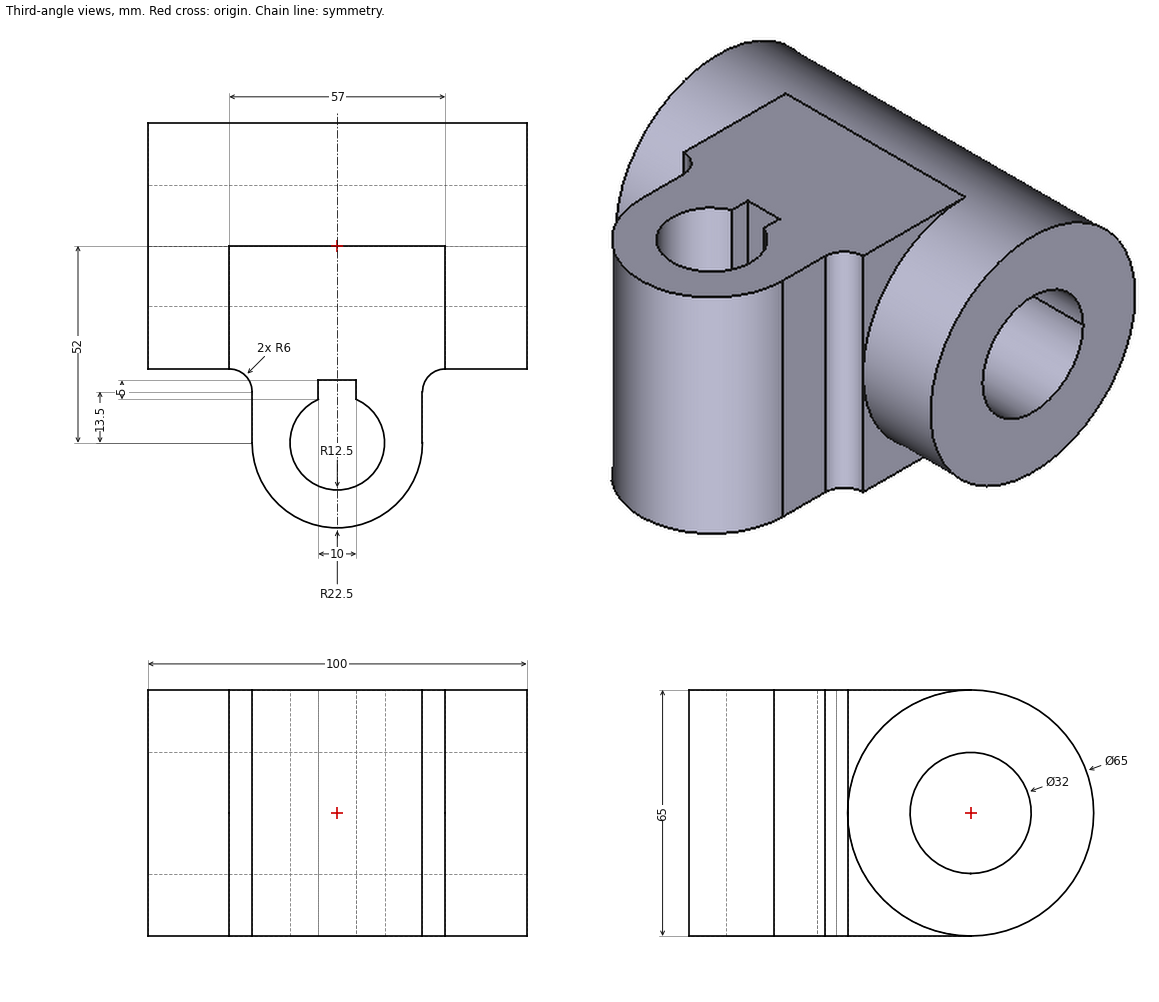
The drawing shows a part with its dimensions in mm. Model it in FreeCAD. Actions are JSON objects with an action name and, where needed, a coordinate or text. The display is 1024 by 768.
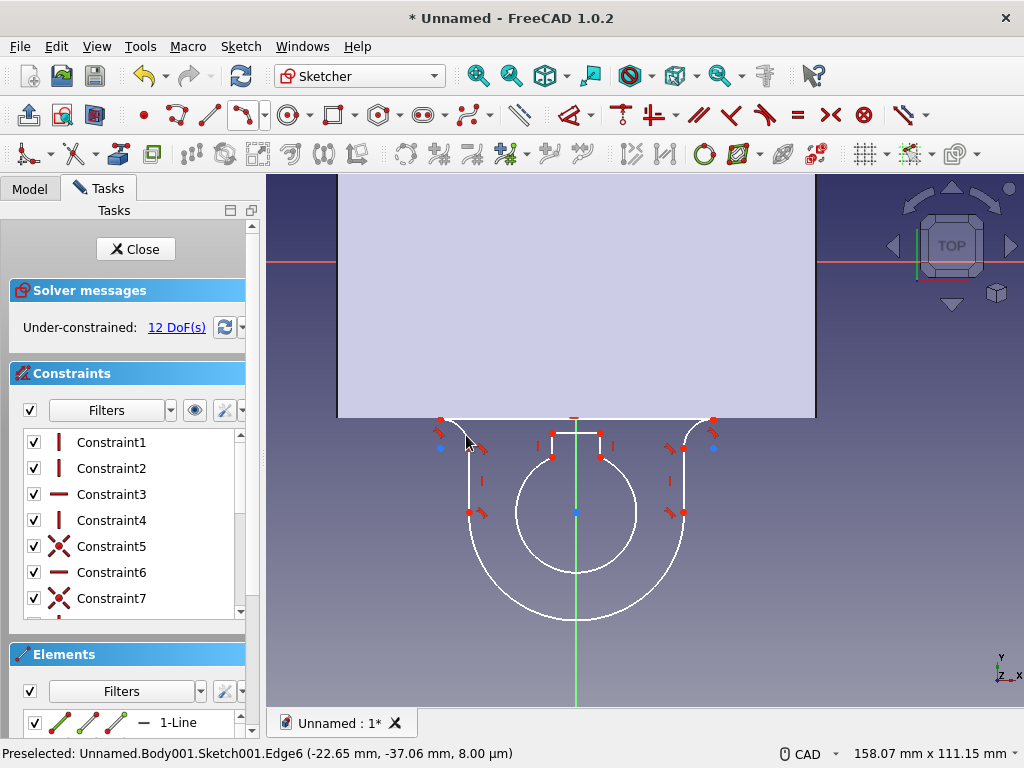
{"action": "left_click", "coordinate": [513, 600]}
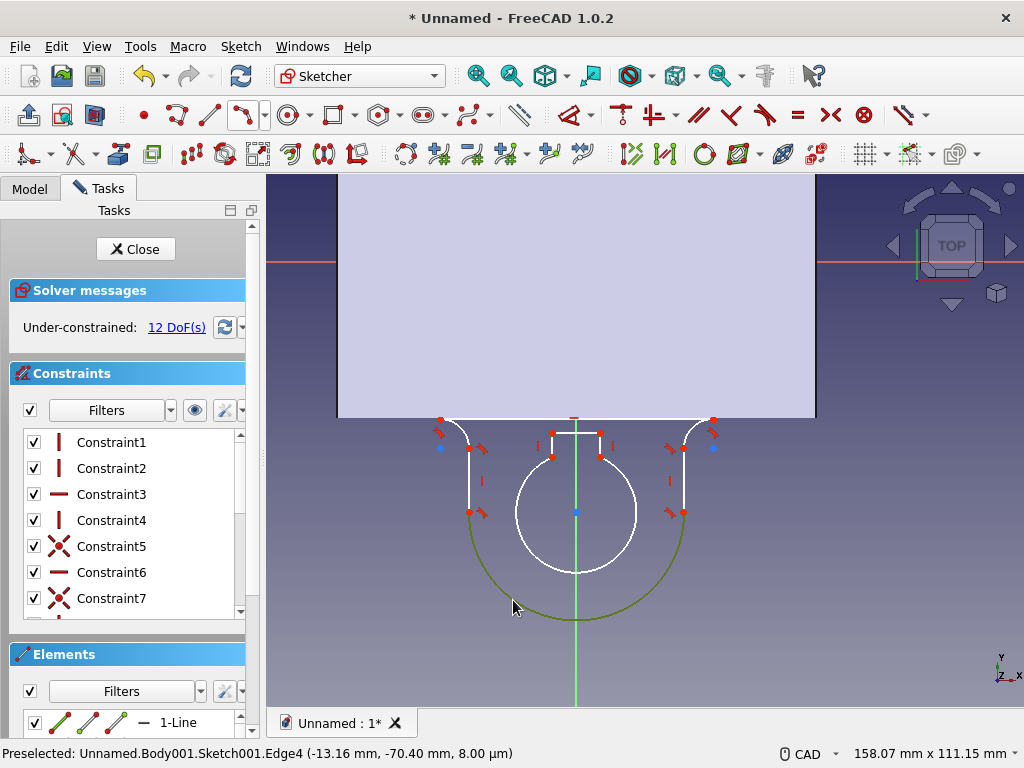
{"action": "left_click", "coordinate": [523, 540]}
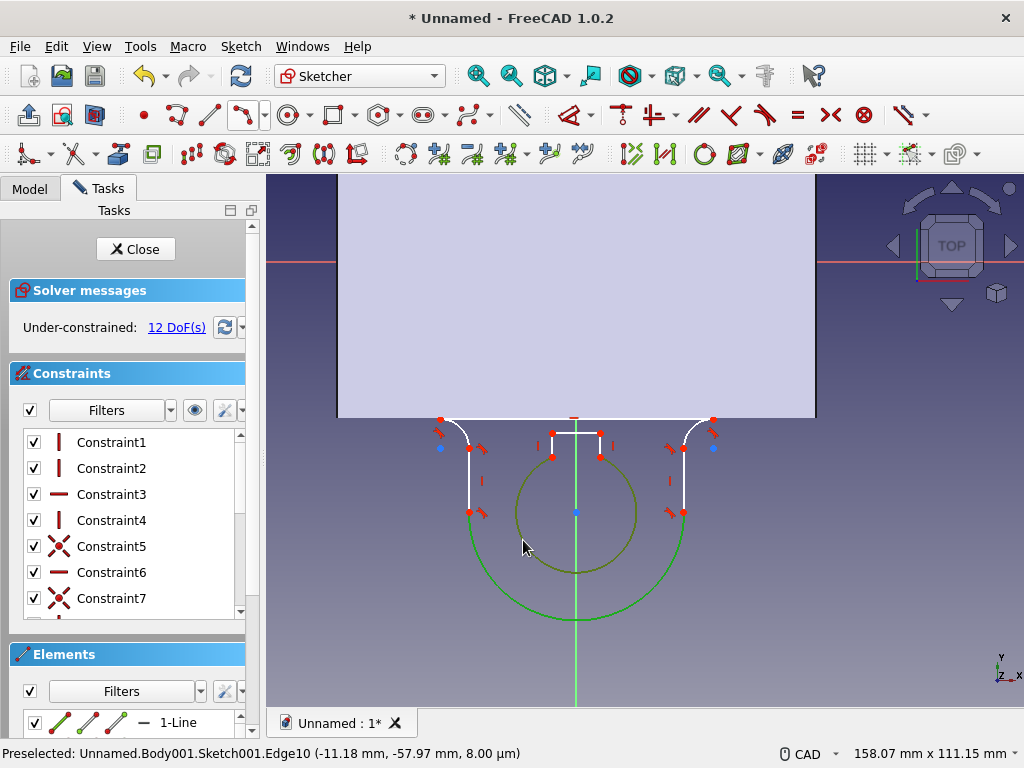
{"action": "key", "text": "c"}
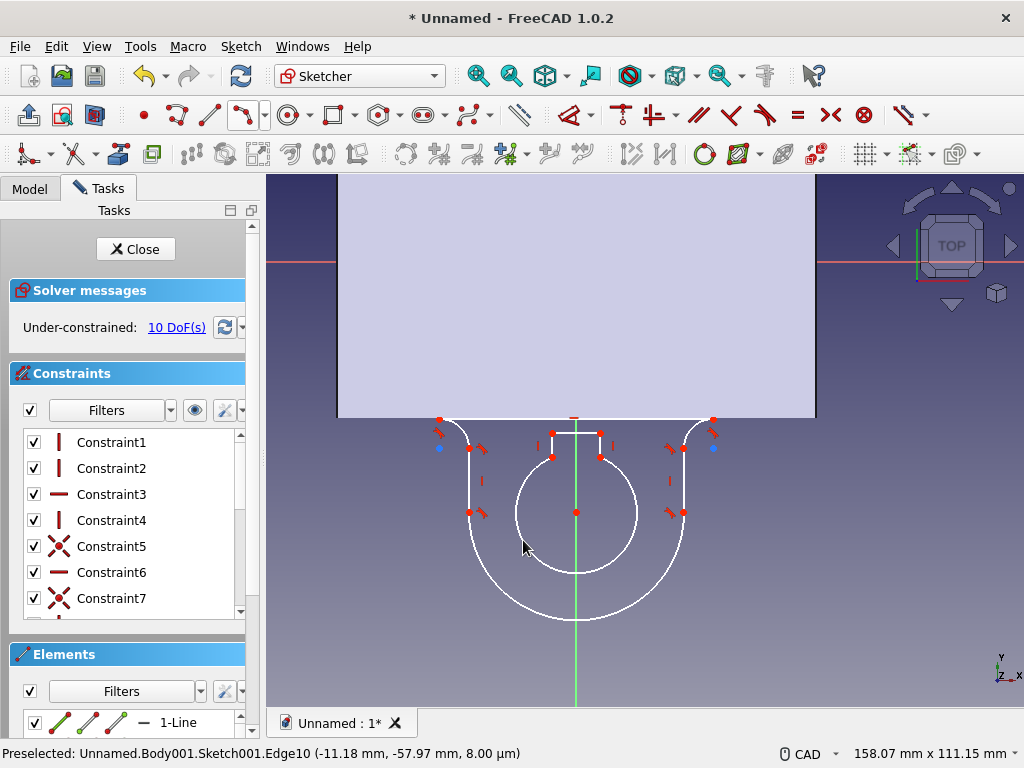
{"action": "left_click", "coordinate": [687, 435]}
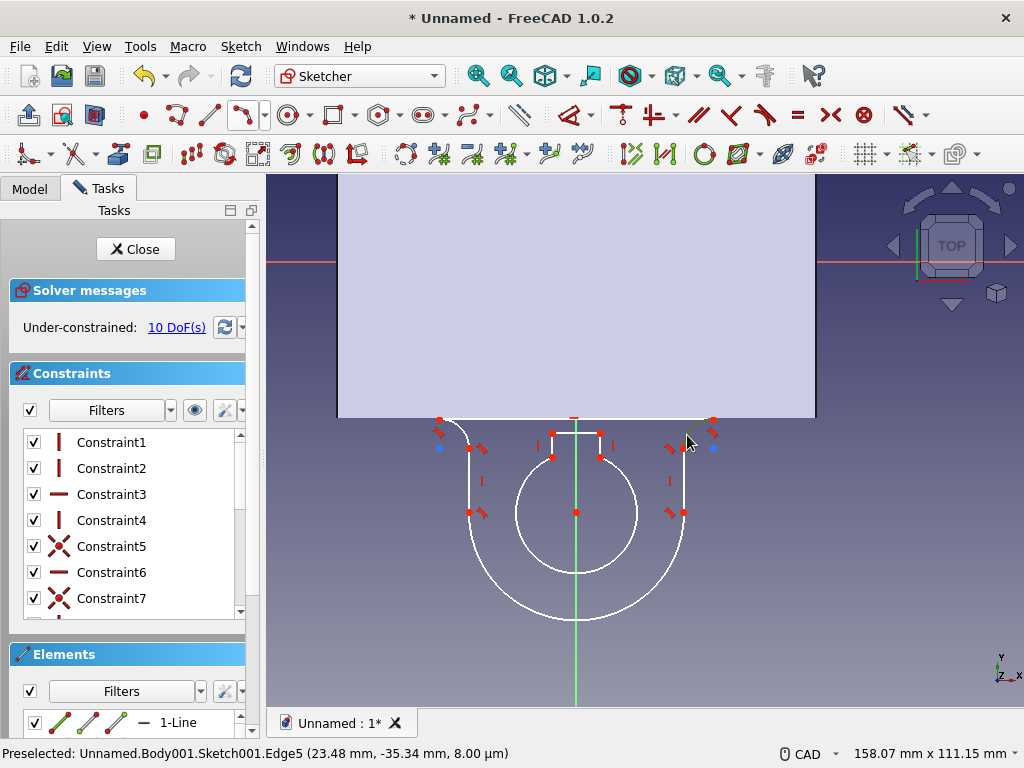
{"action": "left_click", "coordinate": [466, 435]}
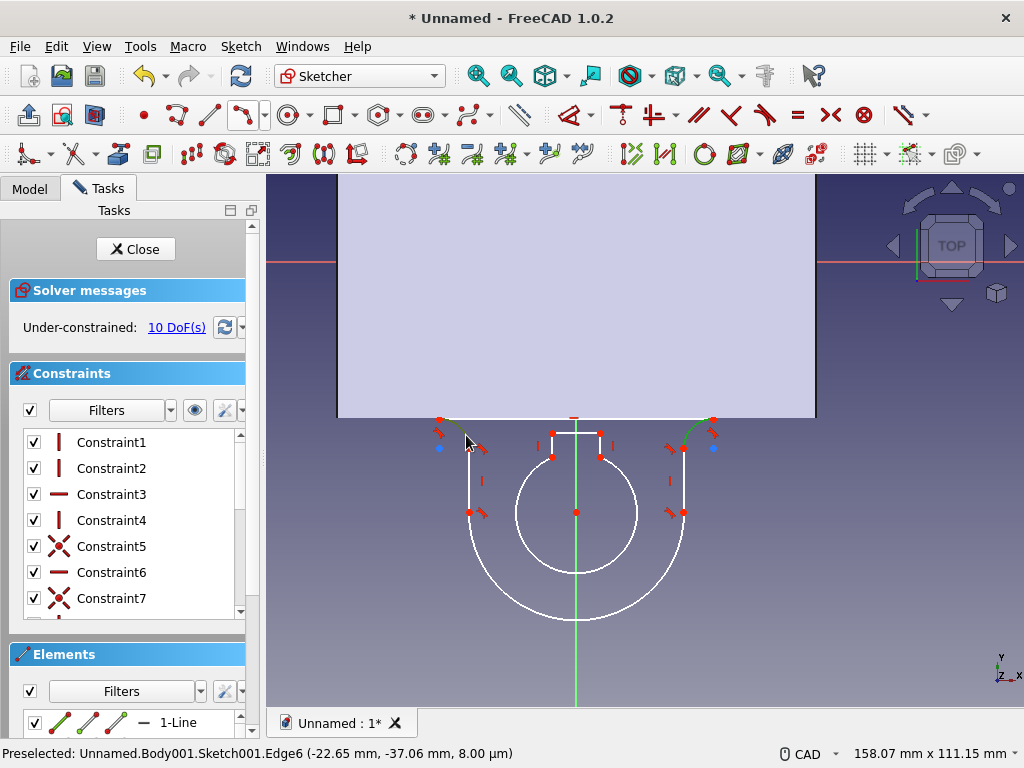
{"action": "key", "text": "e"}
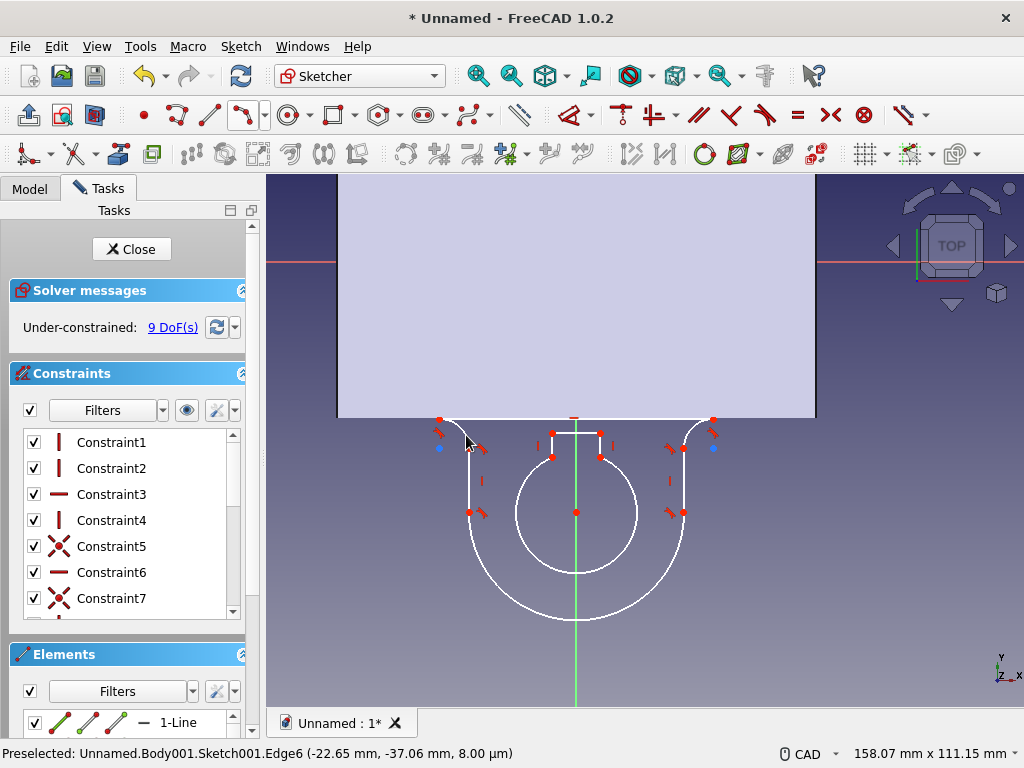
{"action": "left_click", "coordinate": [576, 513]}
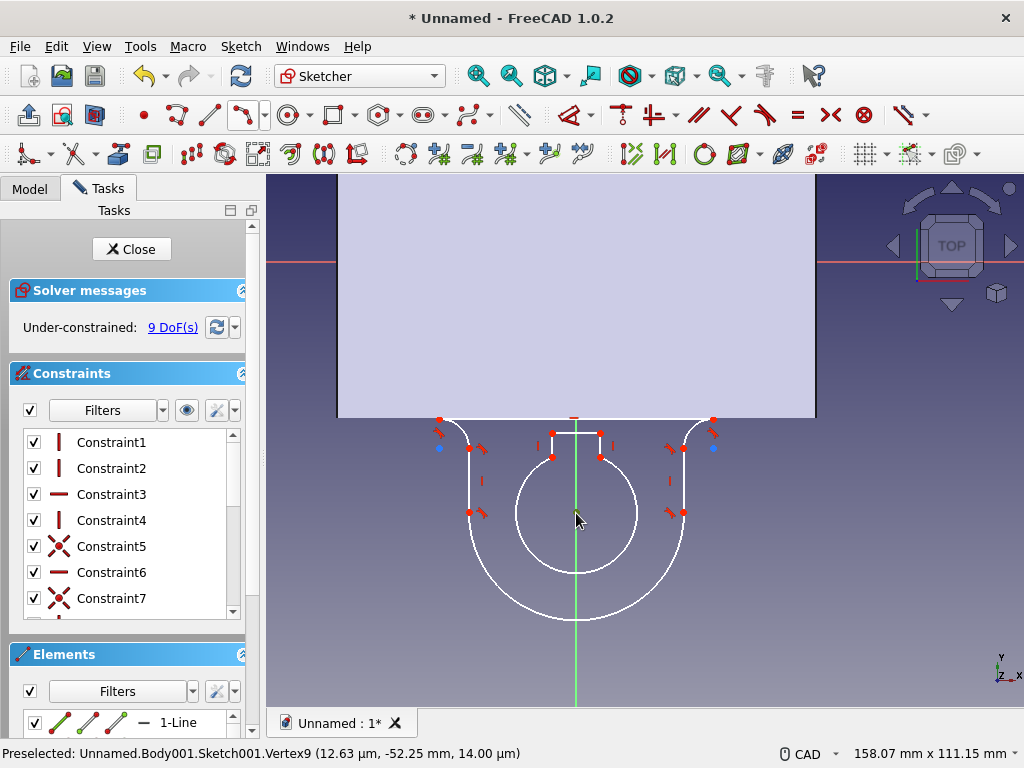
{"action": "left_click", "coordinate": [576, 543]}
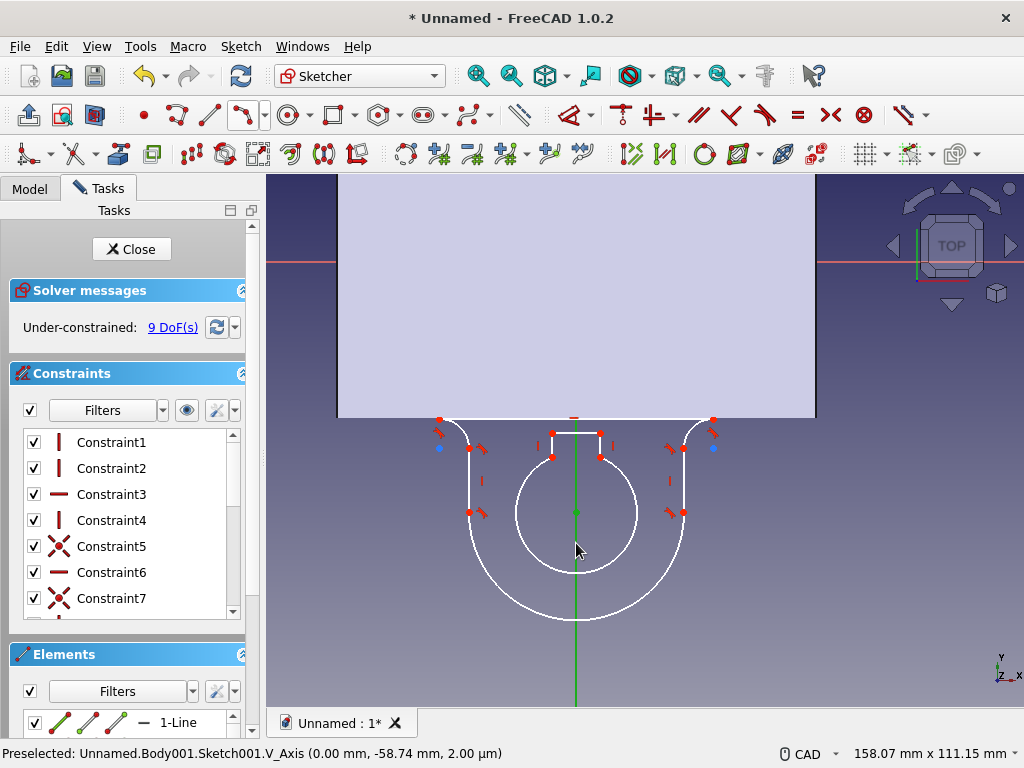
{"action": "left_click", "coordinate": [621, 116]}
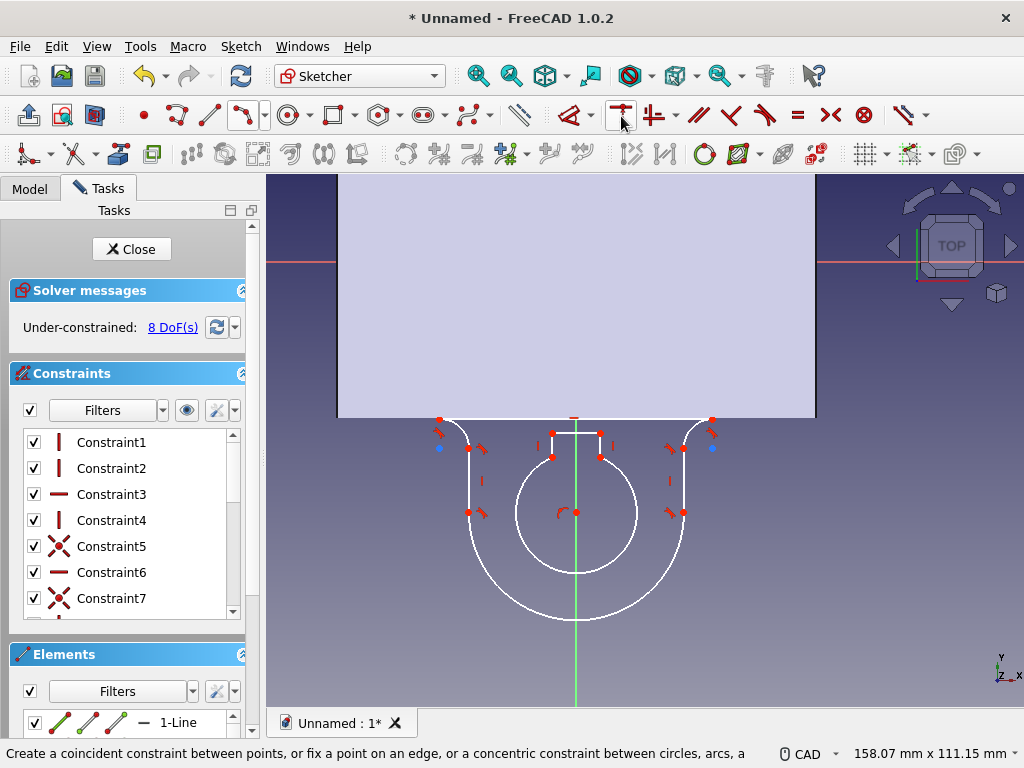
{"action": "left_click", "coordinate": [513, 600]}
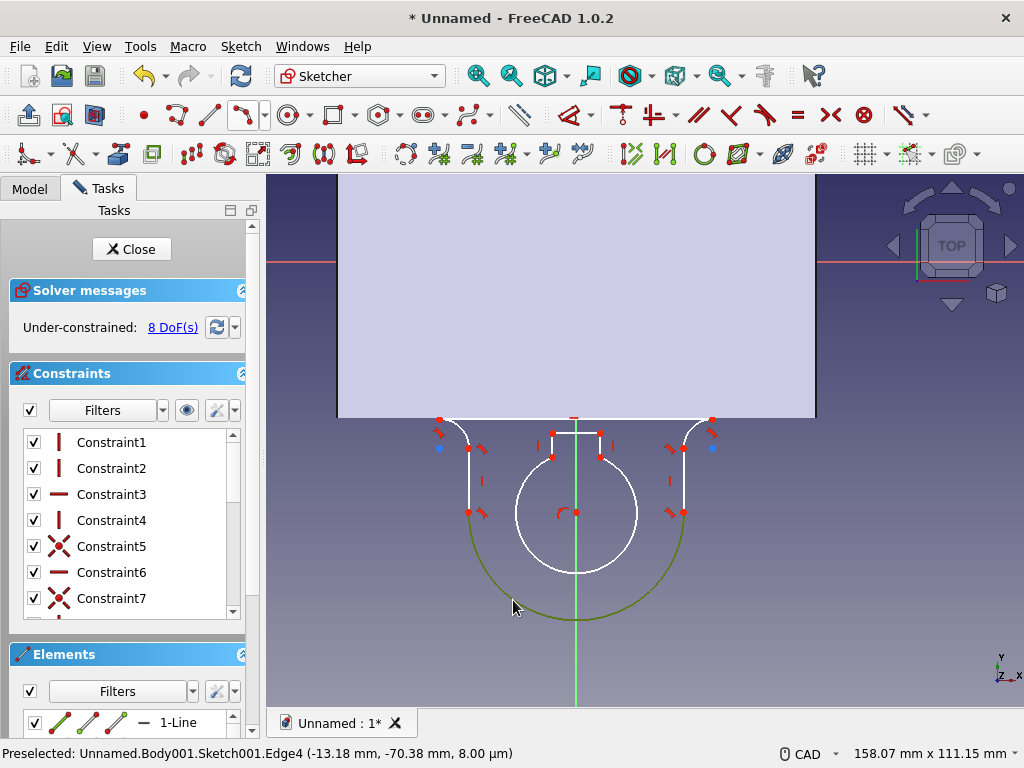
{"action": "key", "text": "k r"}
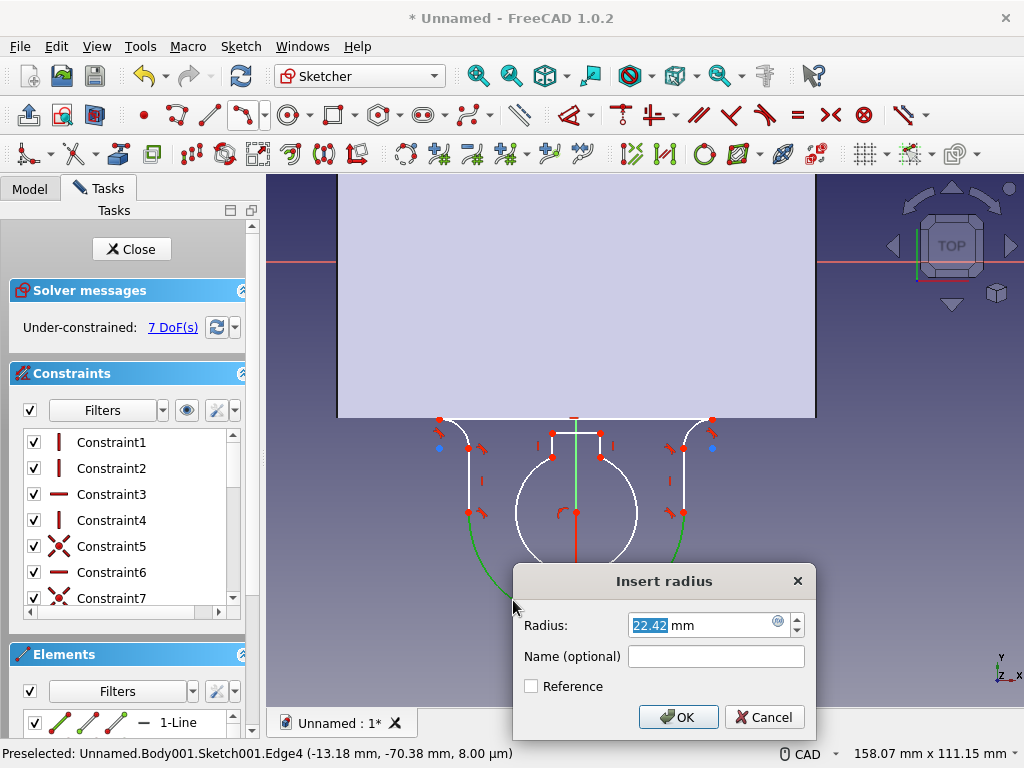
{"action": "type", "text": "22.5"}
{"action": "key", "text": "Return"}